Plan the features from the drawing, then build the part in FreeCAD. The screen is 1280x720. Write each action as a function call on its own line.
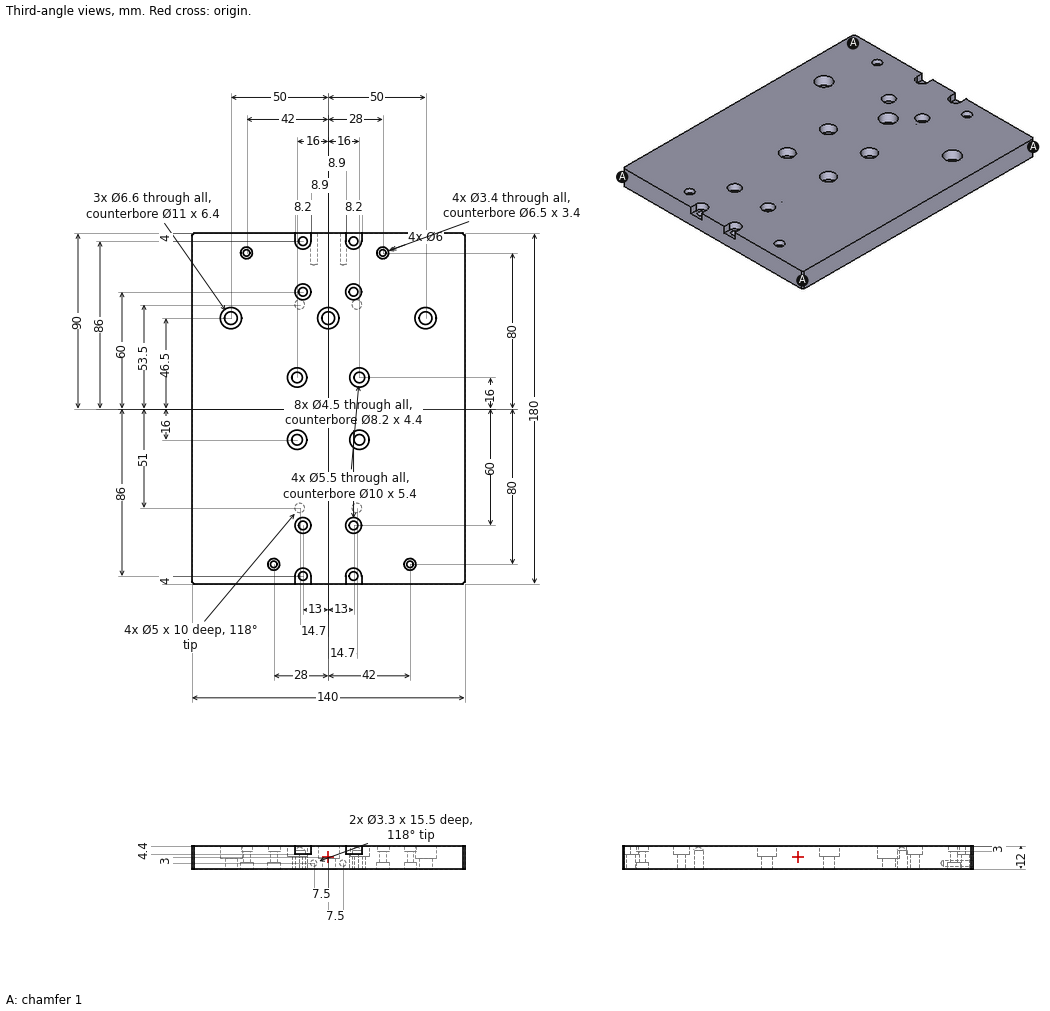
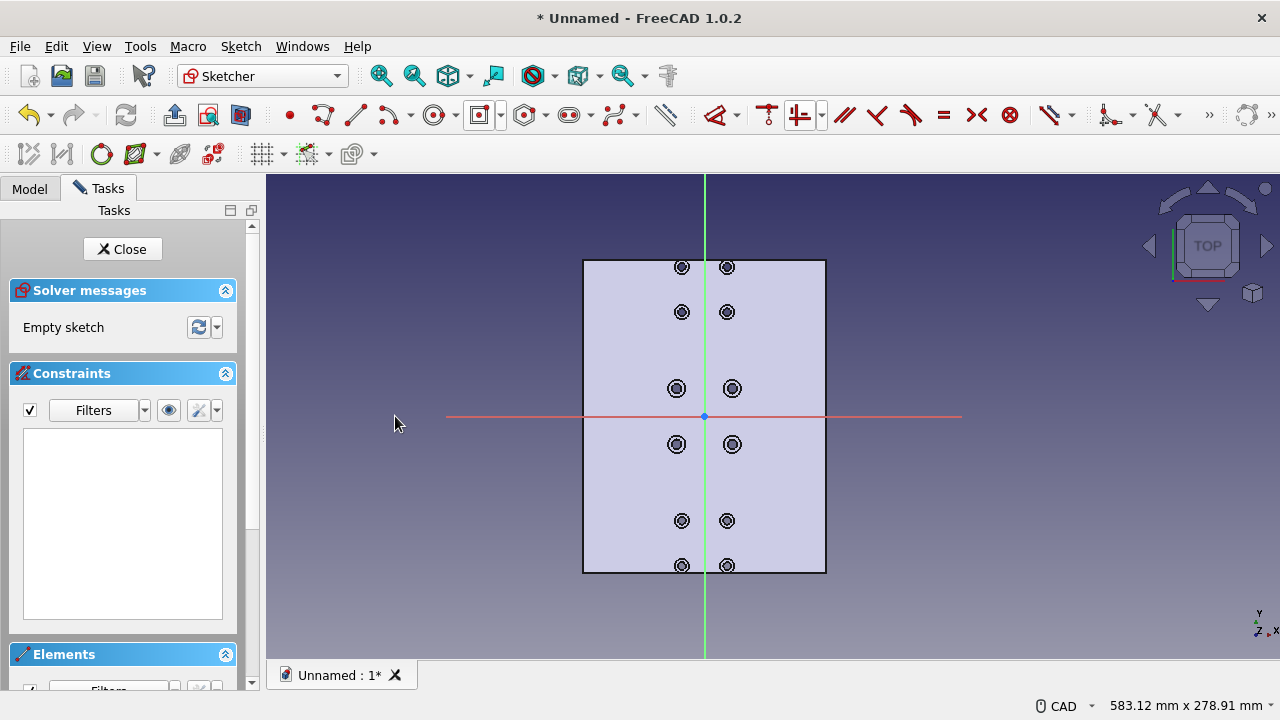
key(g)
key(r)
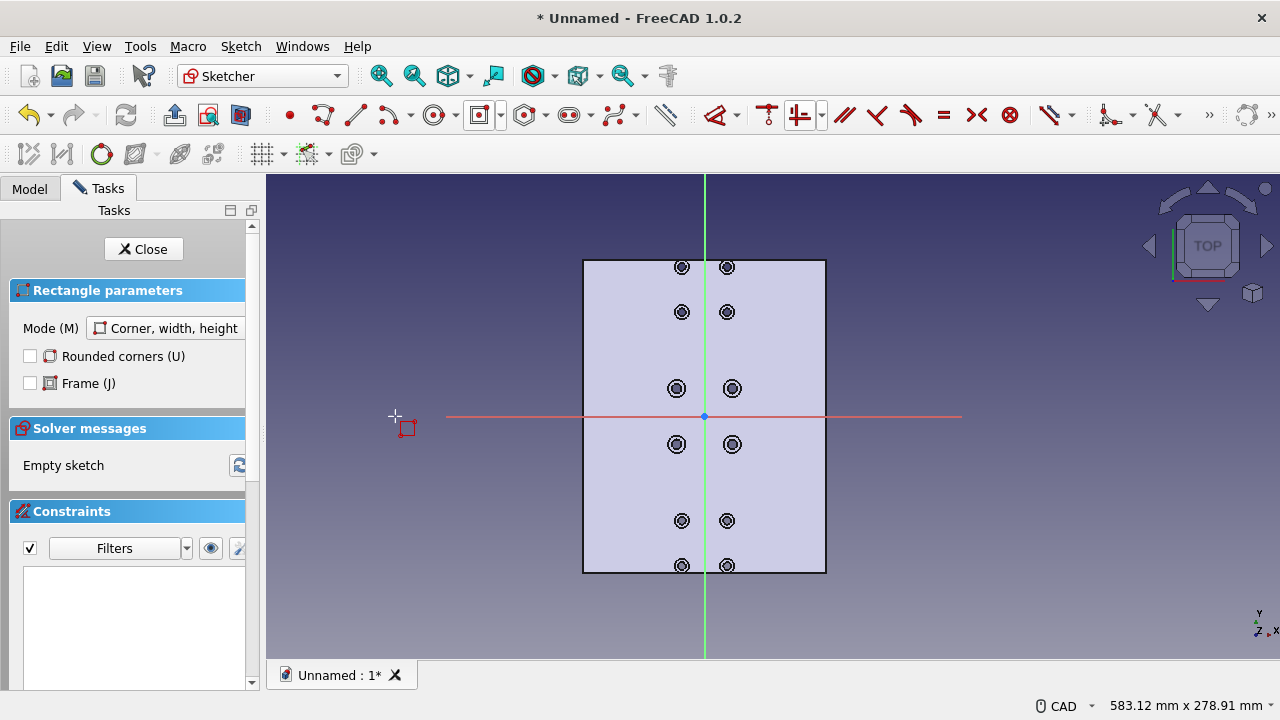
scroll(675, 260, up, 5)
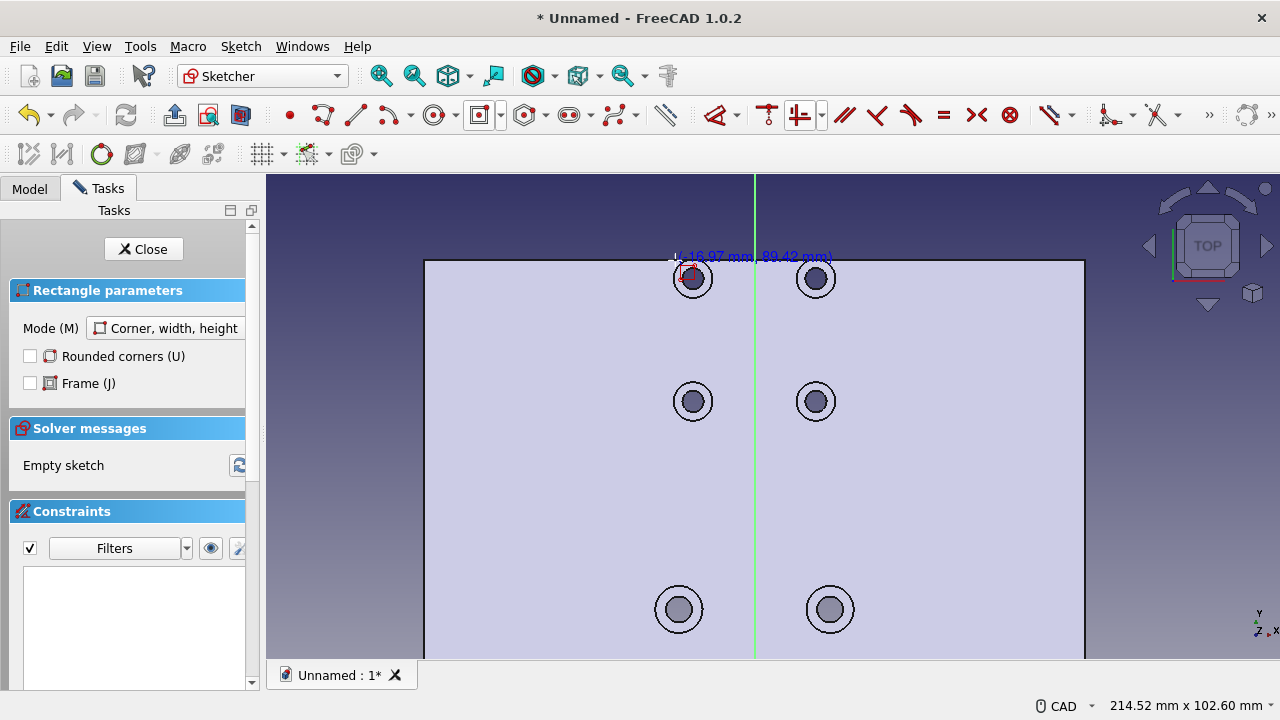
click(674, 260)
click(712, 279)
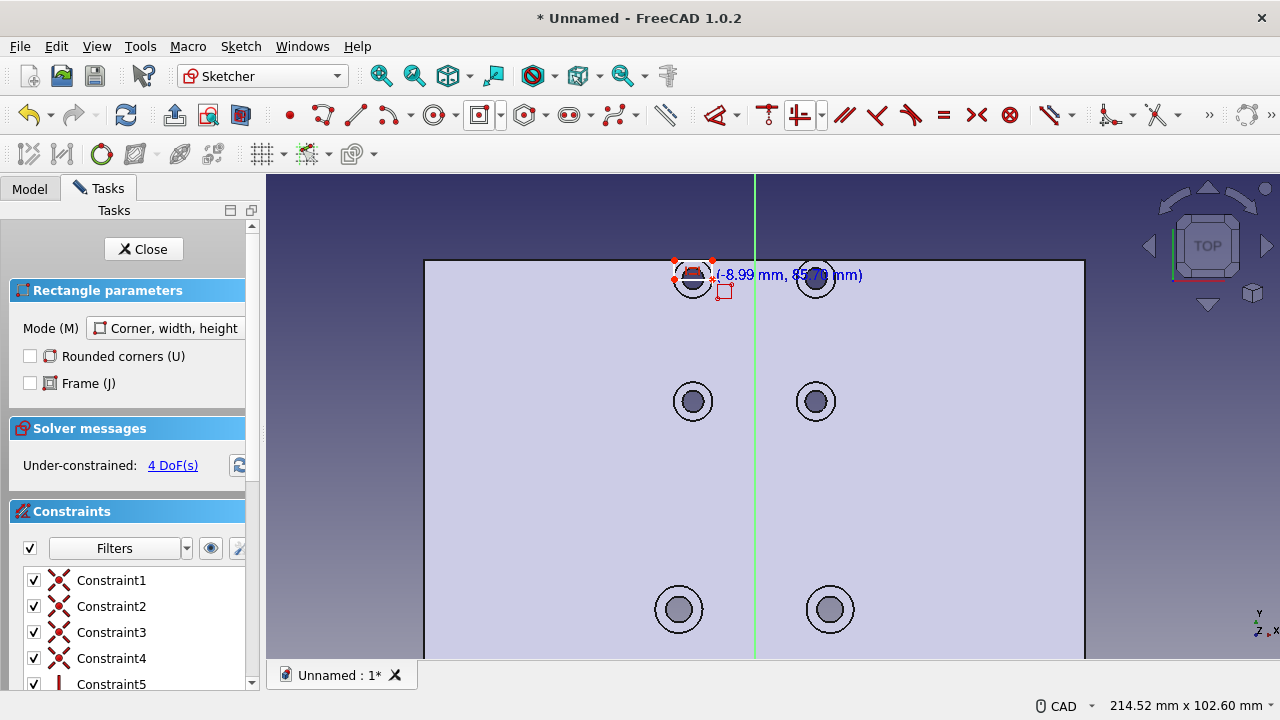
click(797, 260)
click(835, 279)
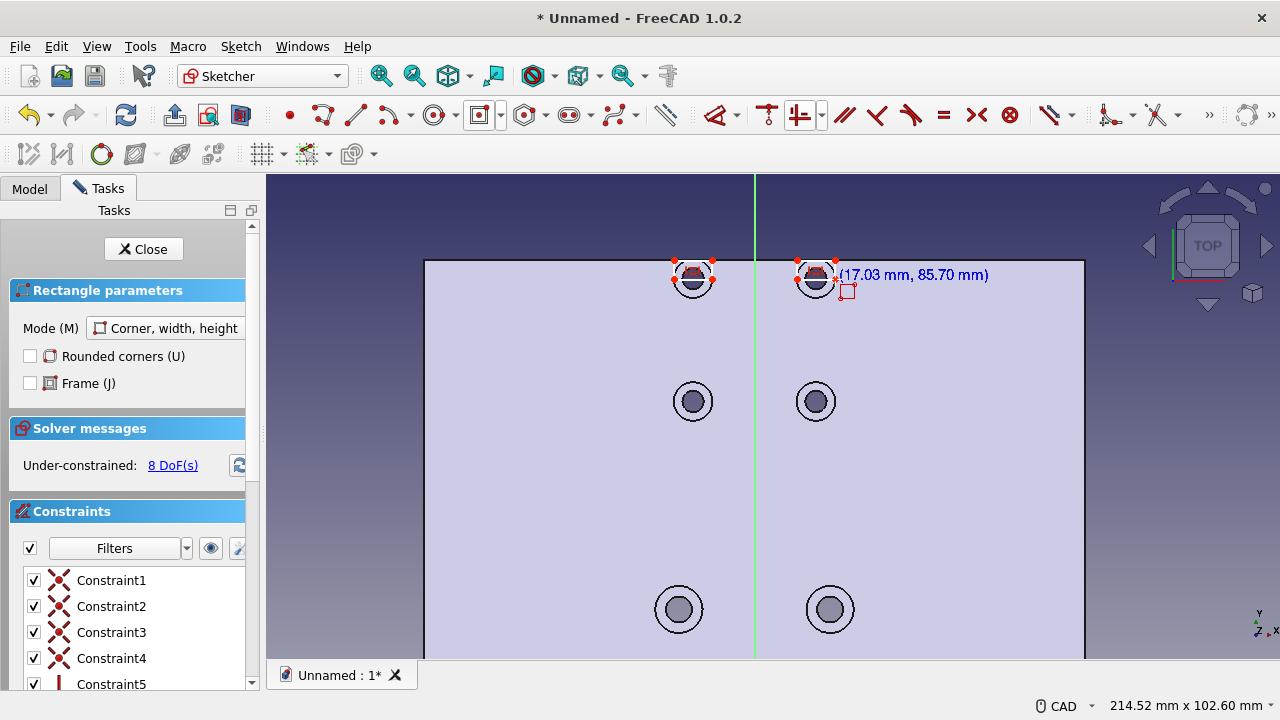
scroll(675, 260, down, 5)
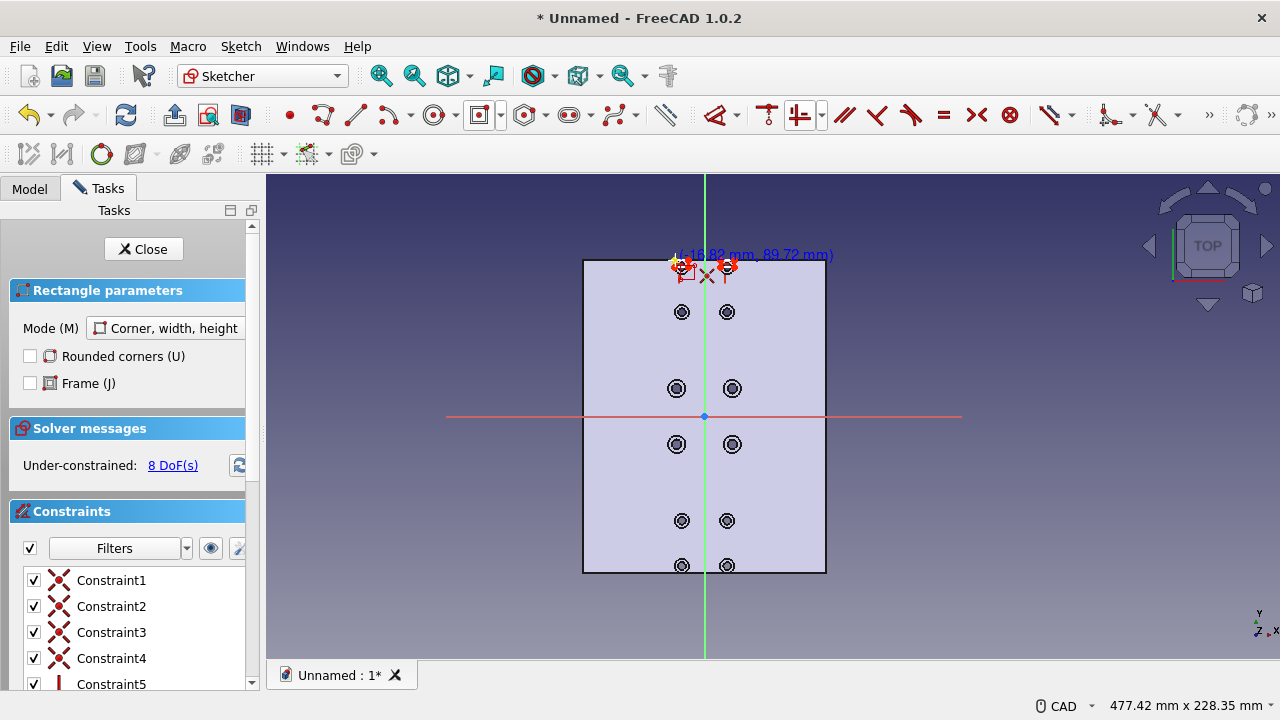
scroll(675, 566, up, 5)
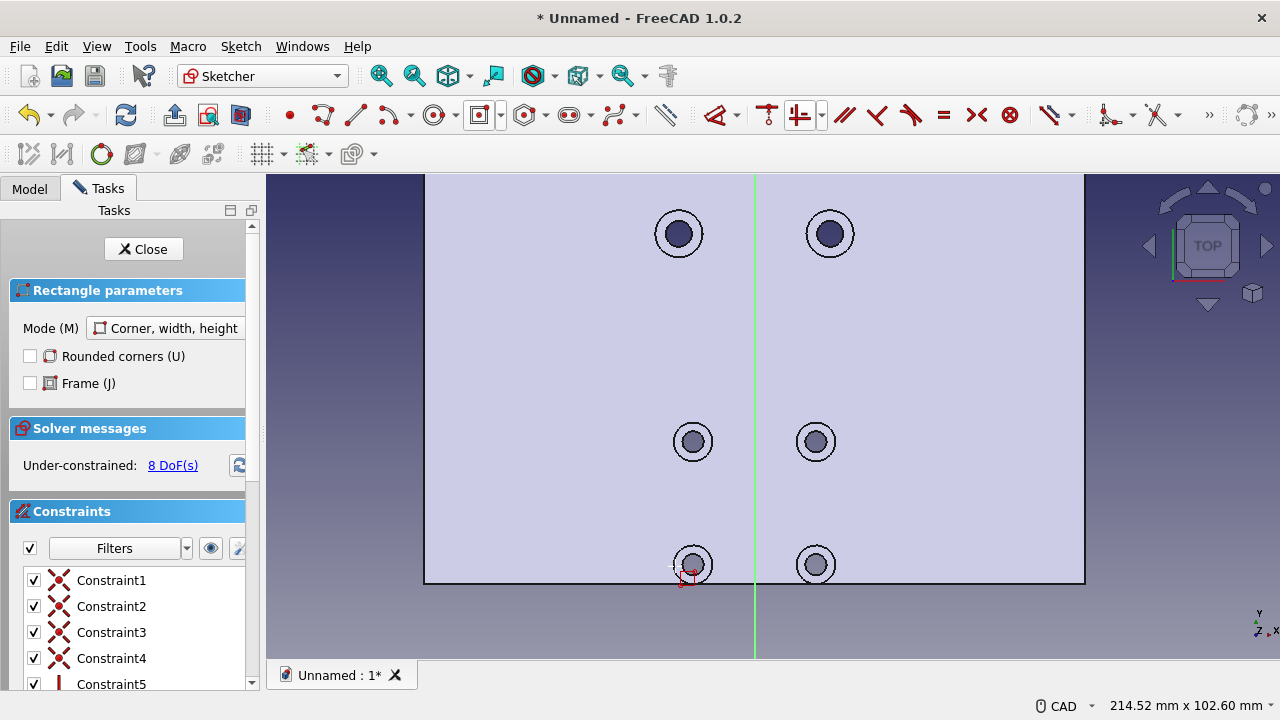
click(674, 565)
click(712, 584)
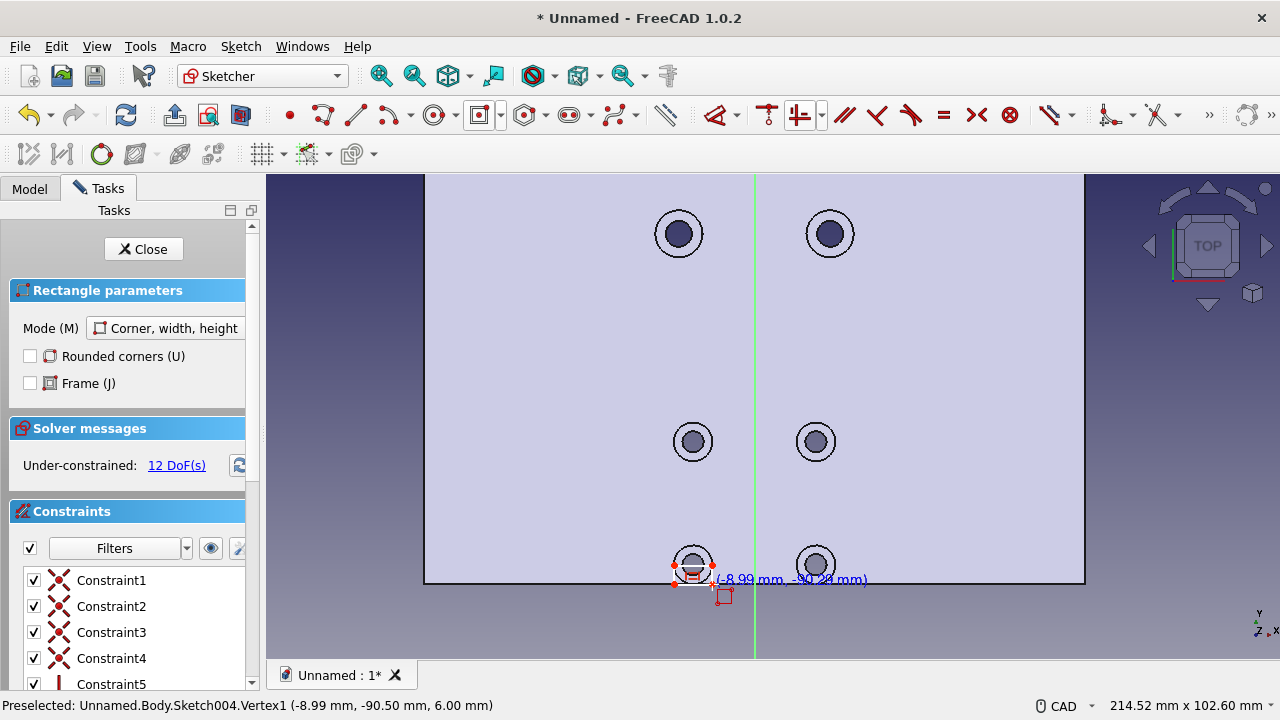
click(797, 565)
click(835, 584)
key(Escape)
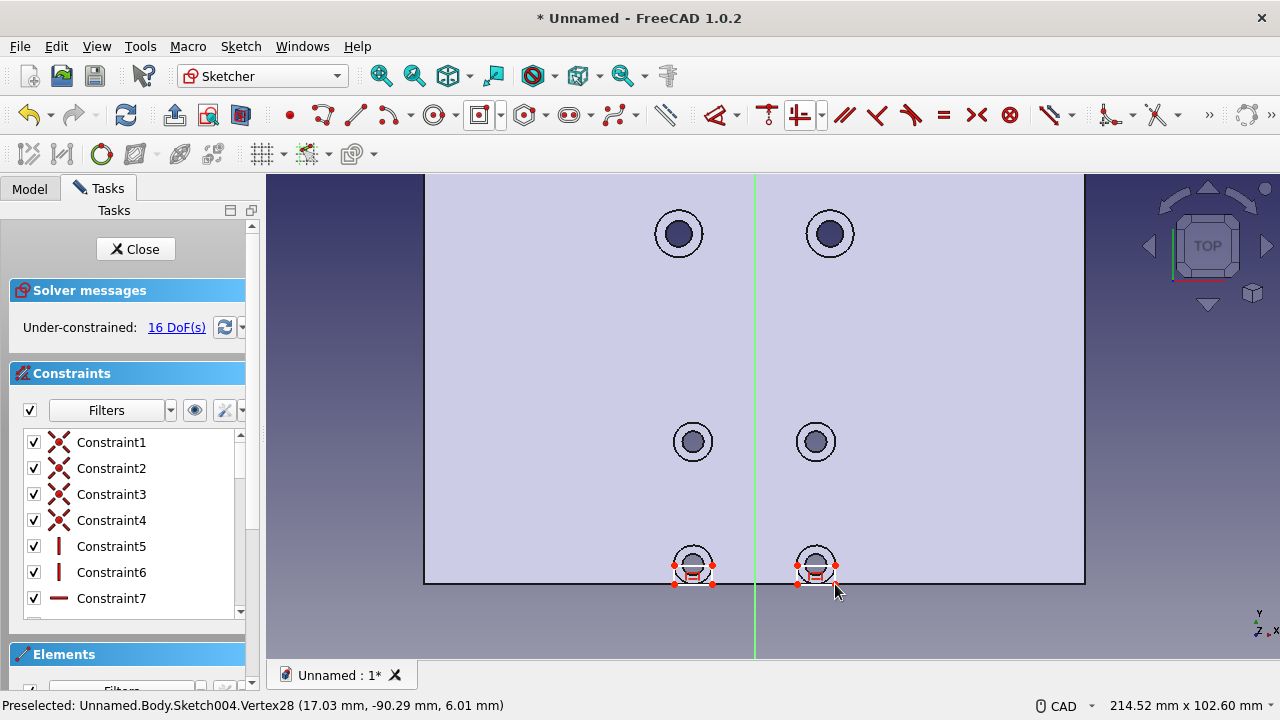
click(714, 116)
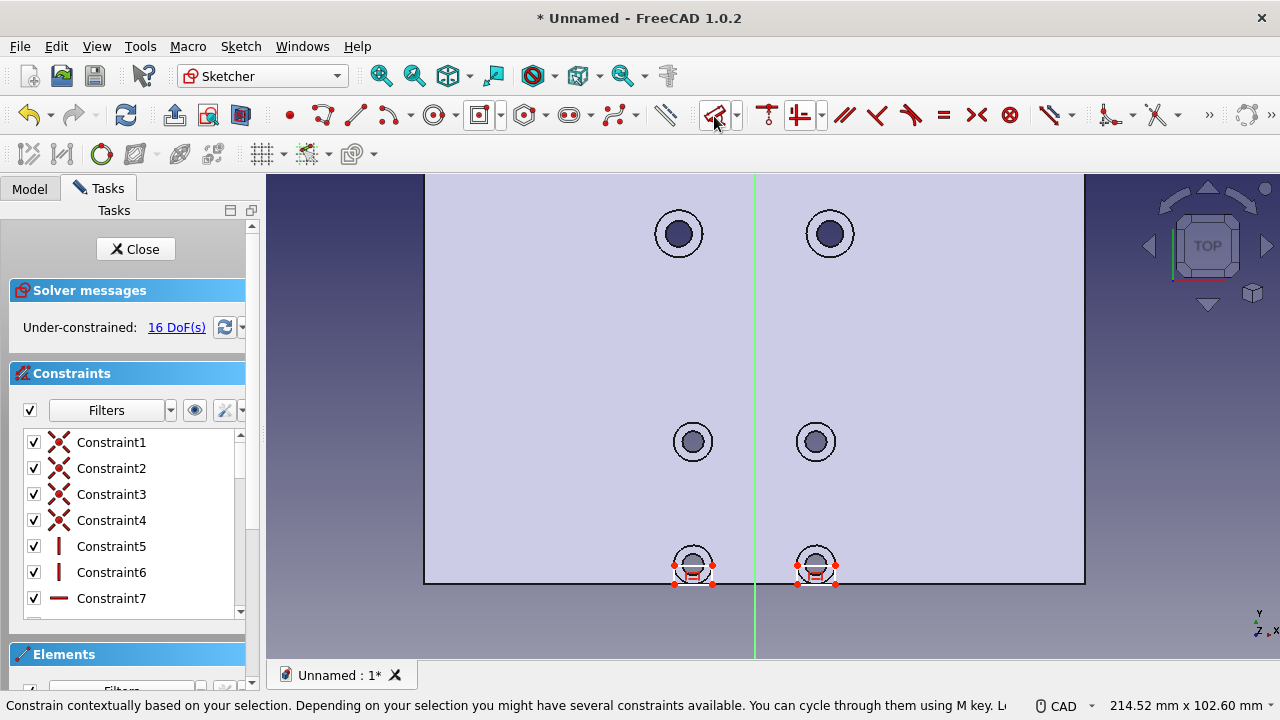
scroll(675, 567, down, 5)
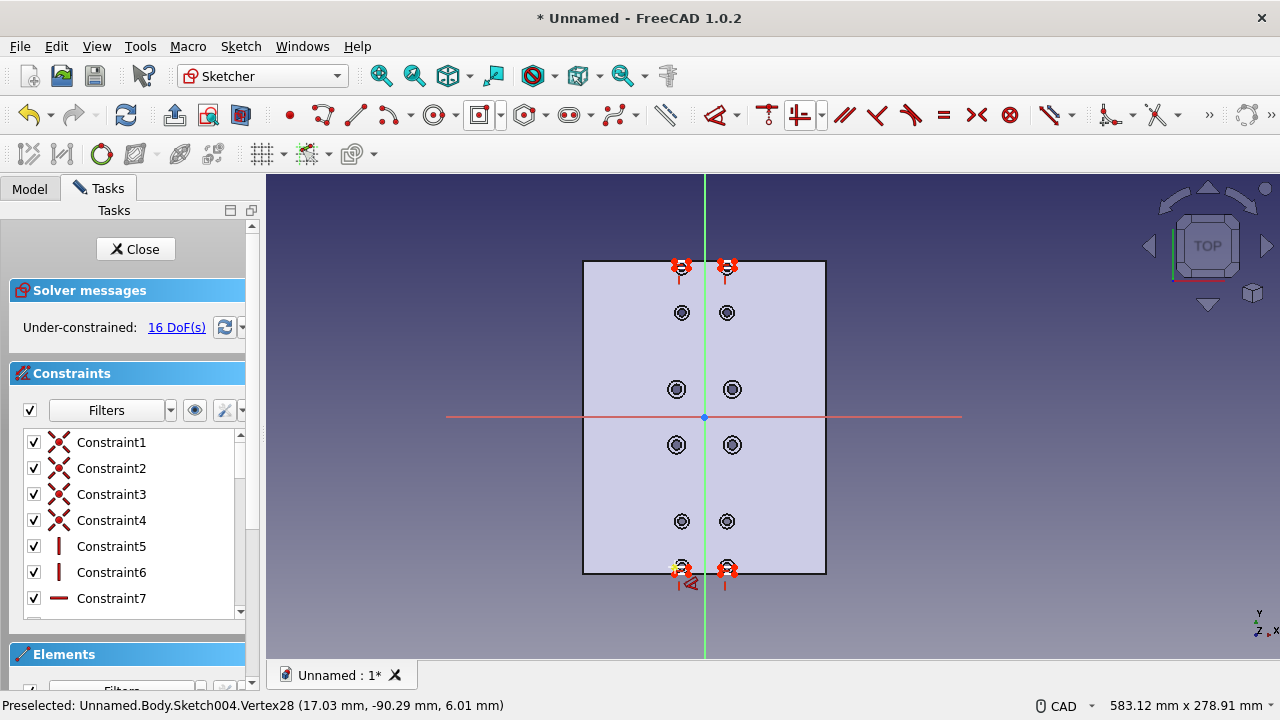
scroll(675, 265, up, 9)